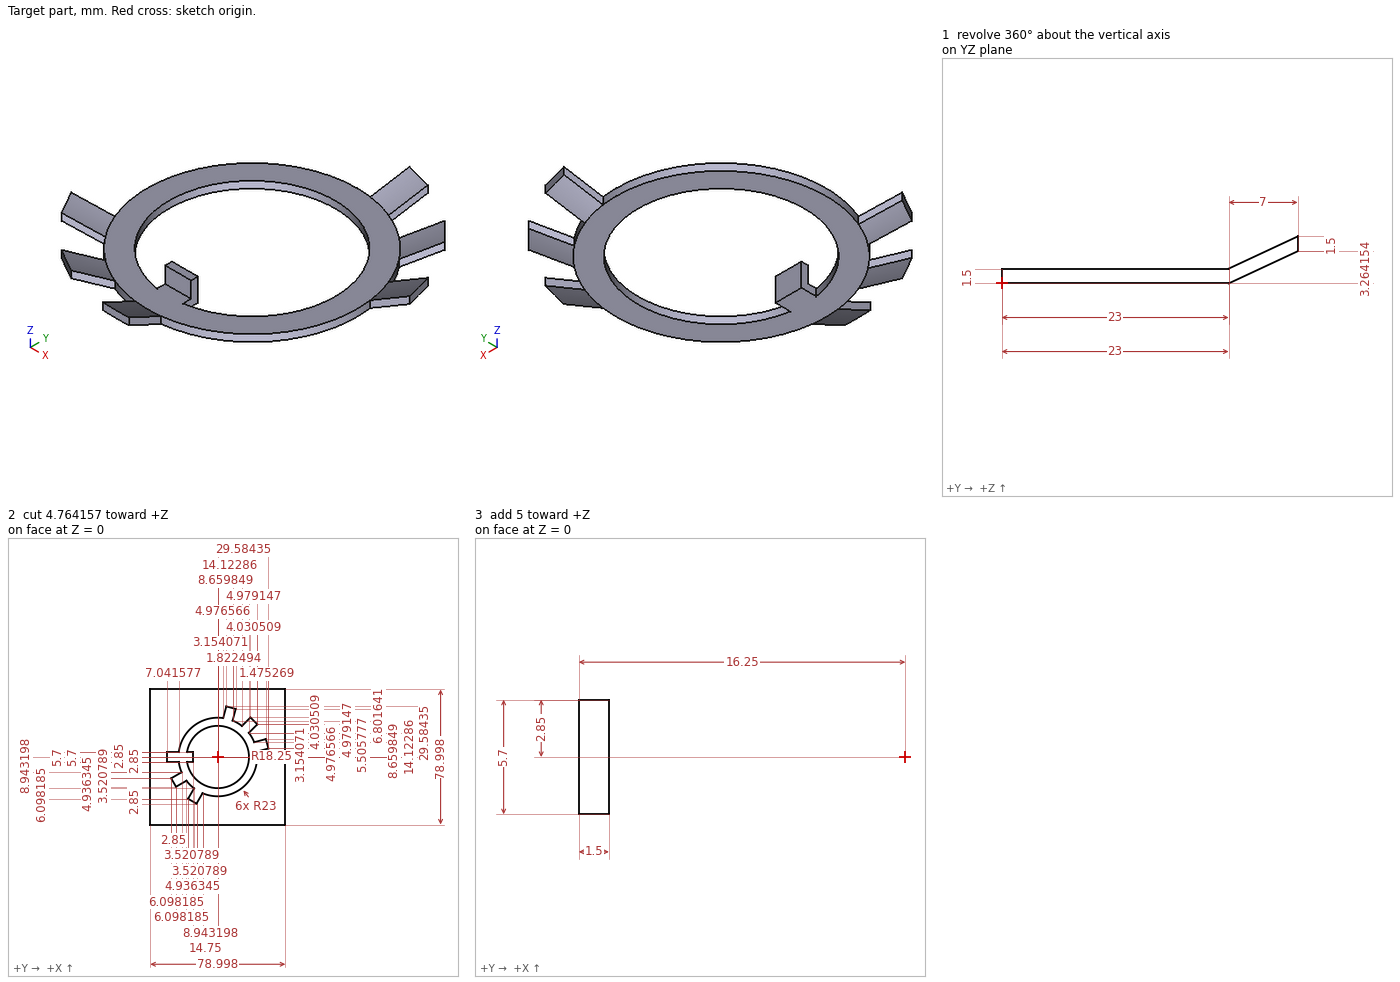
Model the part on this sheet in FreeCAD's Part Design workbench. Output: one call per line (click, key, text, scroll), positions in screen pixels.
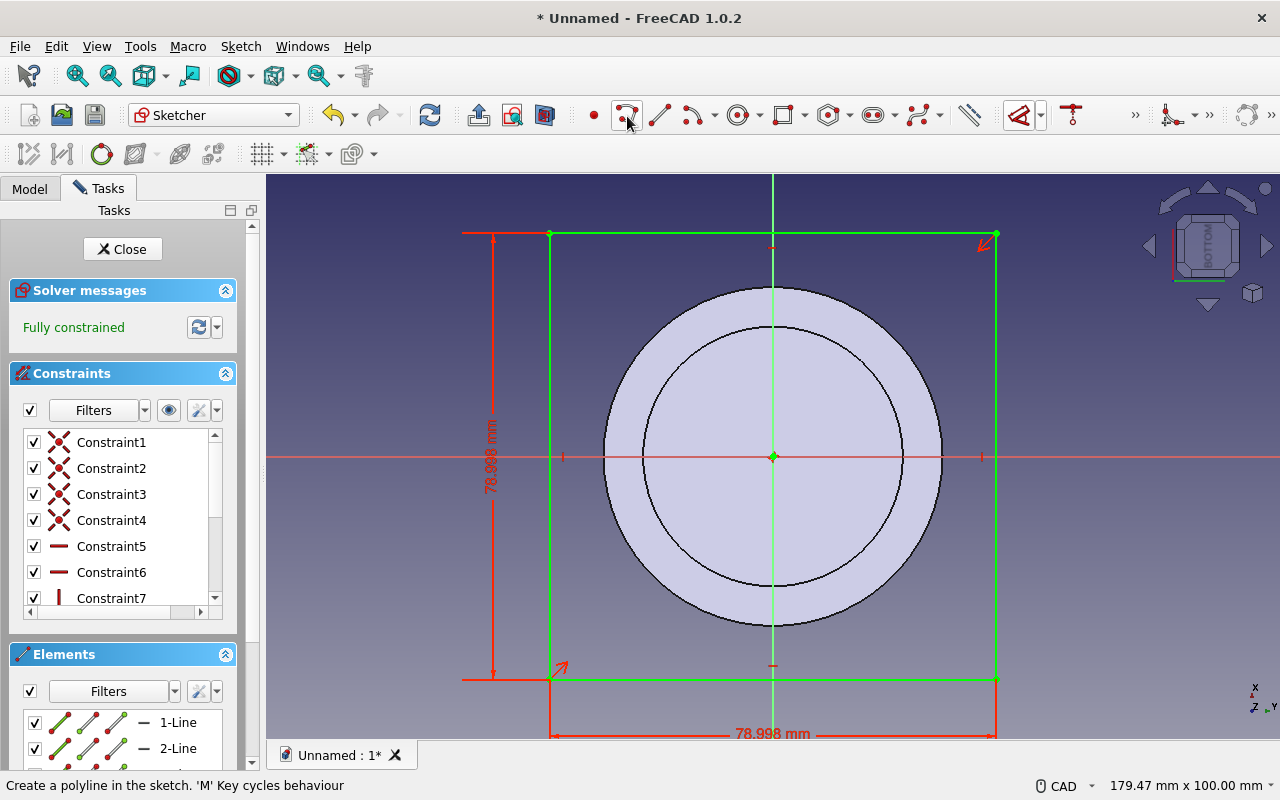
click(671, 473)
click(690, 473)
click(690, 440)
click(671, 440)
right_click(671, 440)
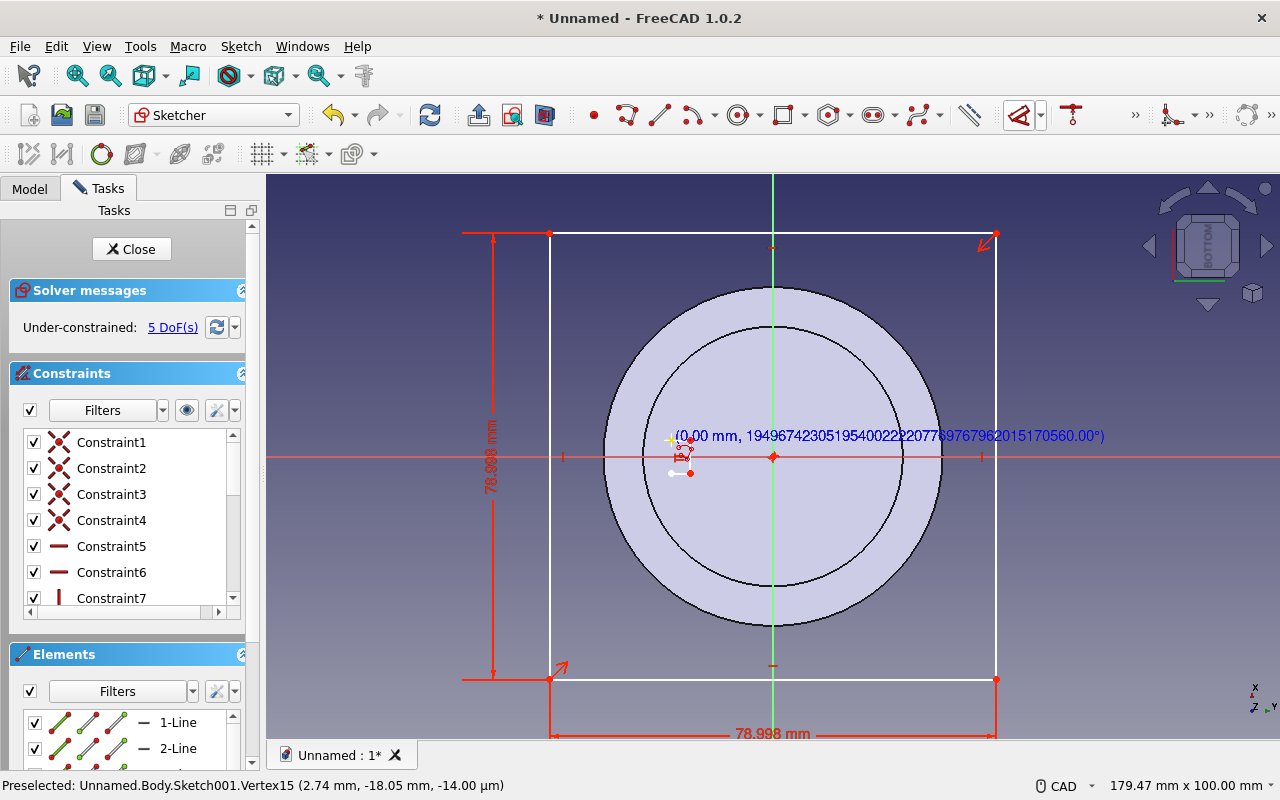
click(714, 116)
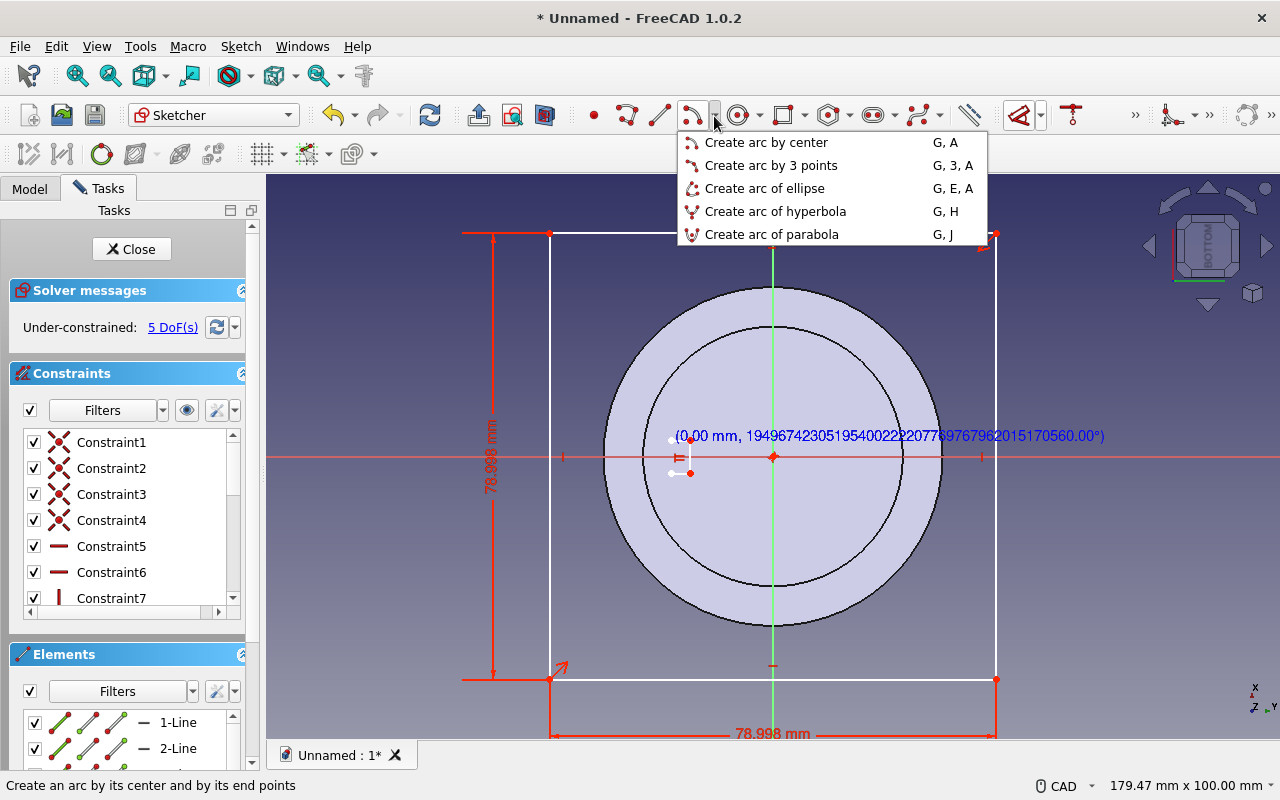
click(832, 166)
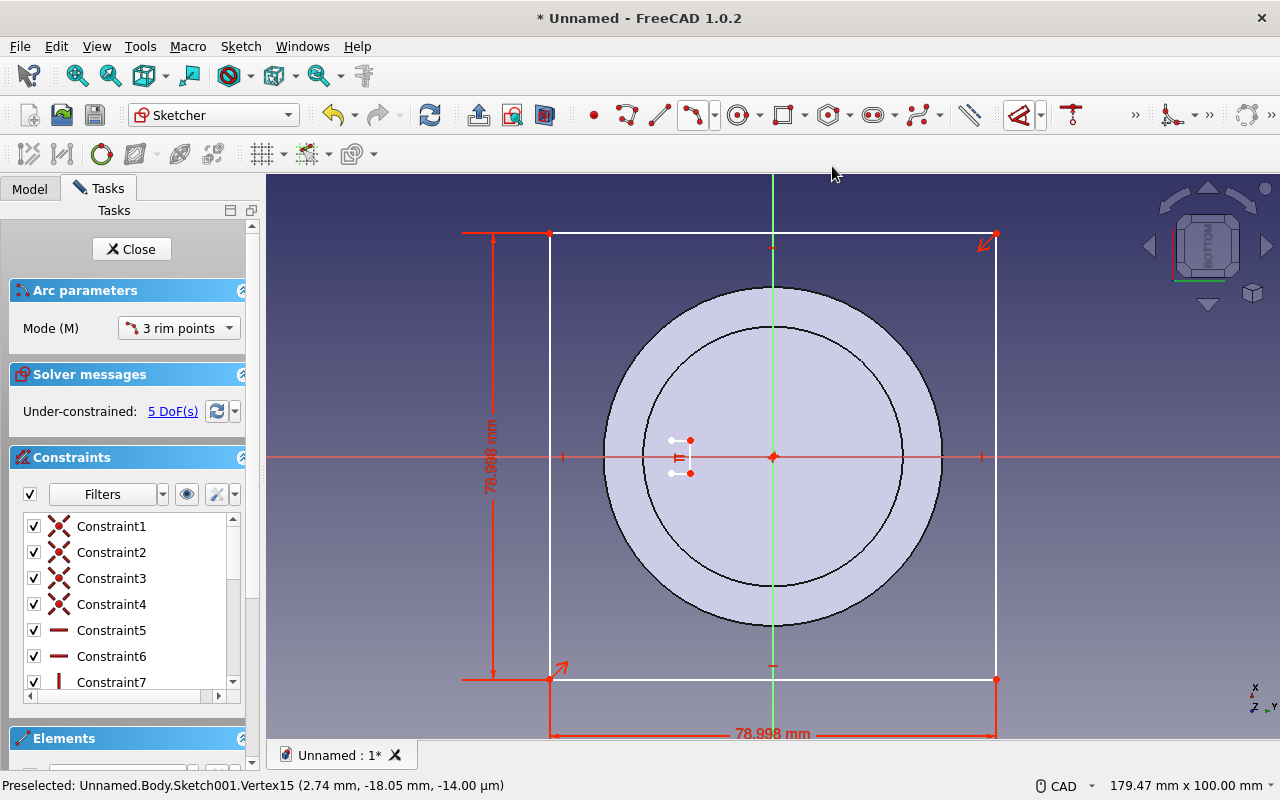
scroll(671, 440, up, 3)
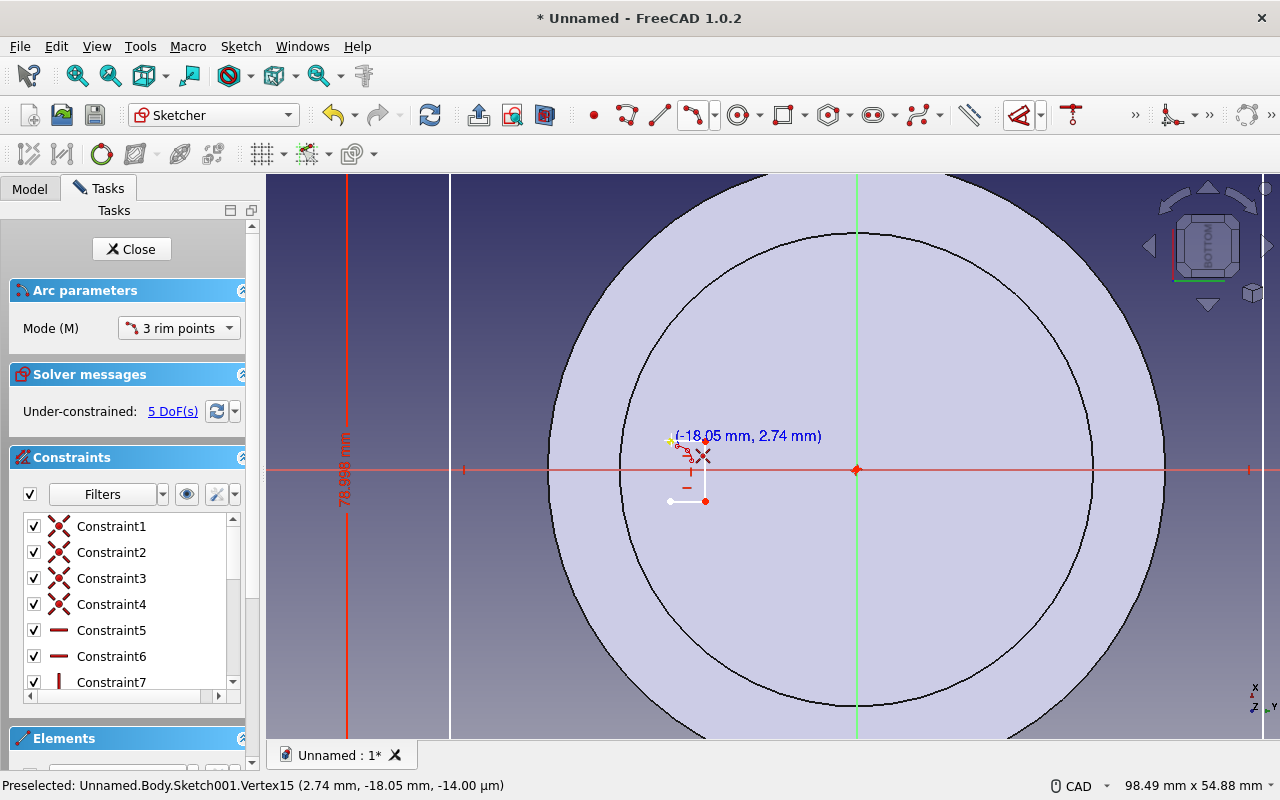
click(671, 441)
click(671, 502)
click(1012, 575)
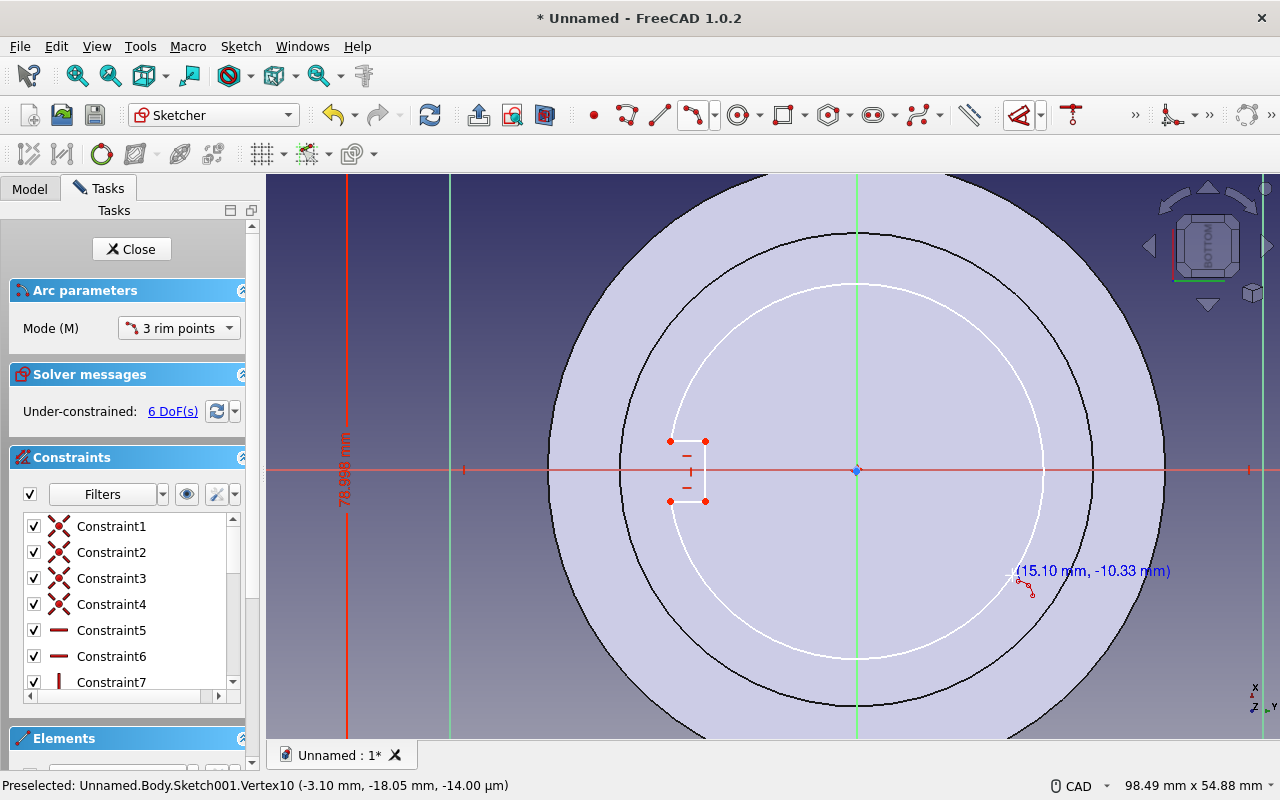
key(g)
key(m)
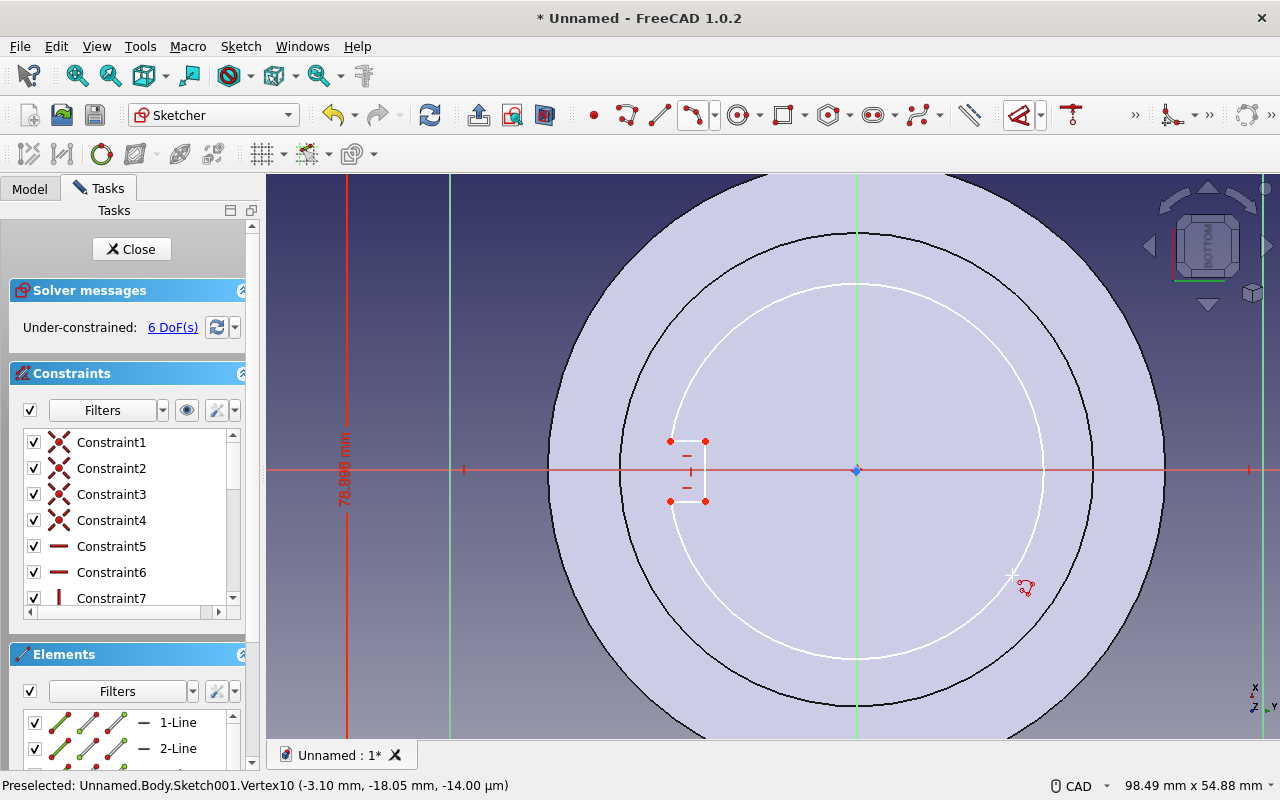
click(638, 562)
click(576, 598)
click(605, 649)
click(668, 613)
right_click(668, 613)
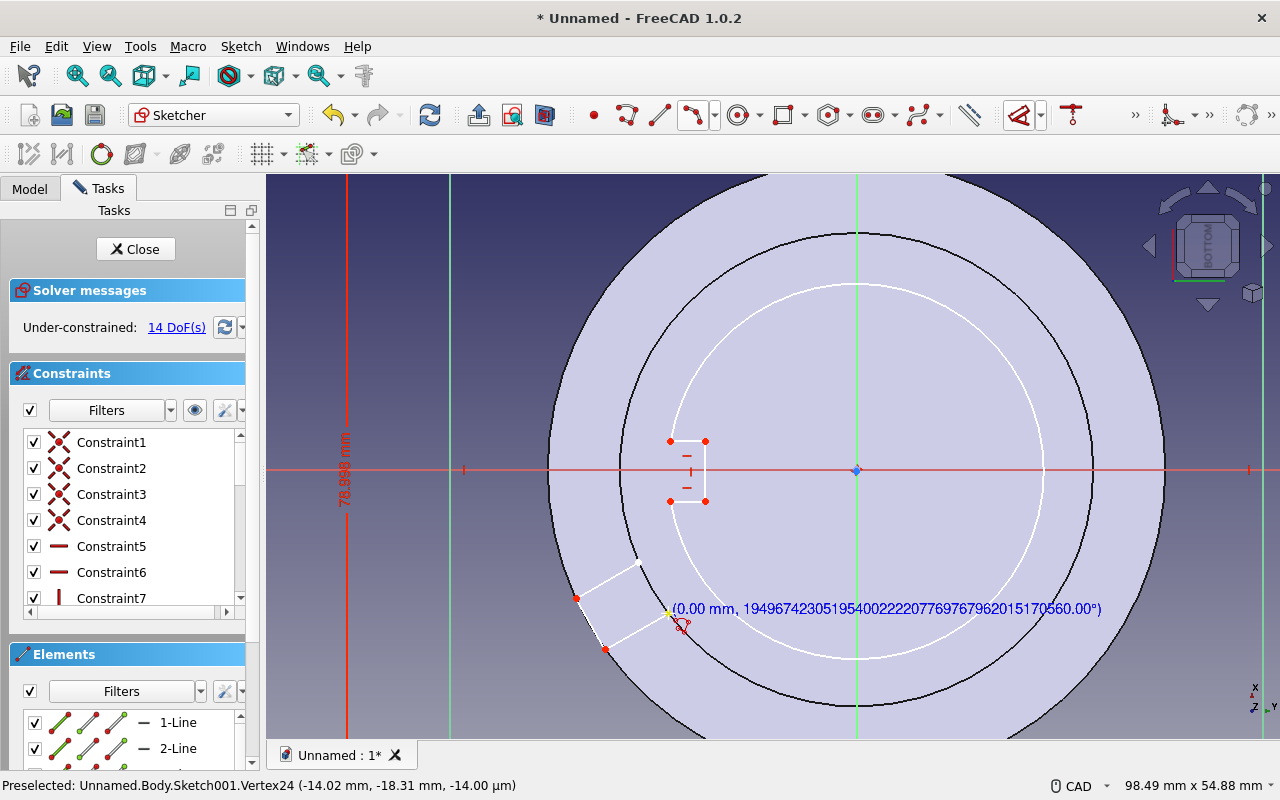
click(714, 658)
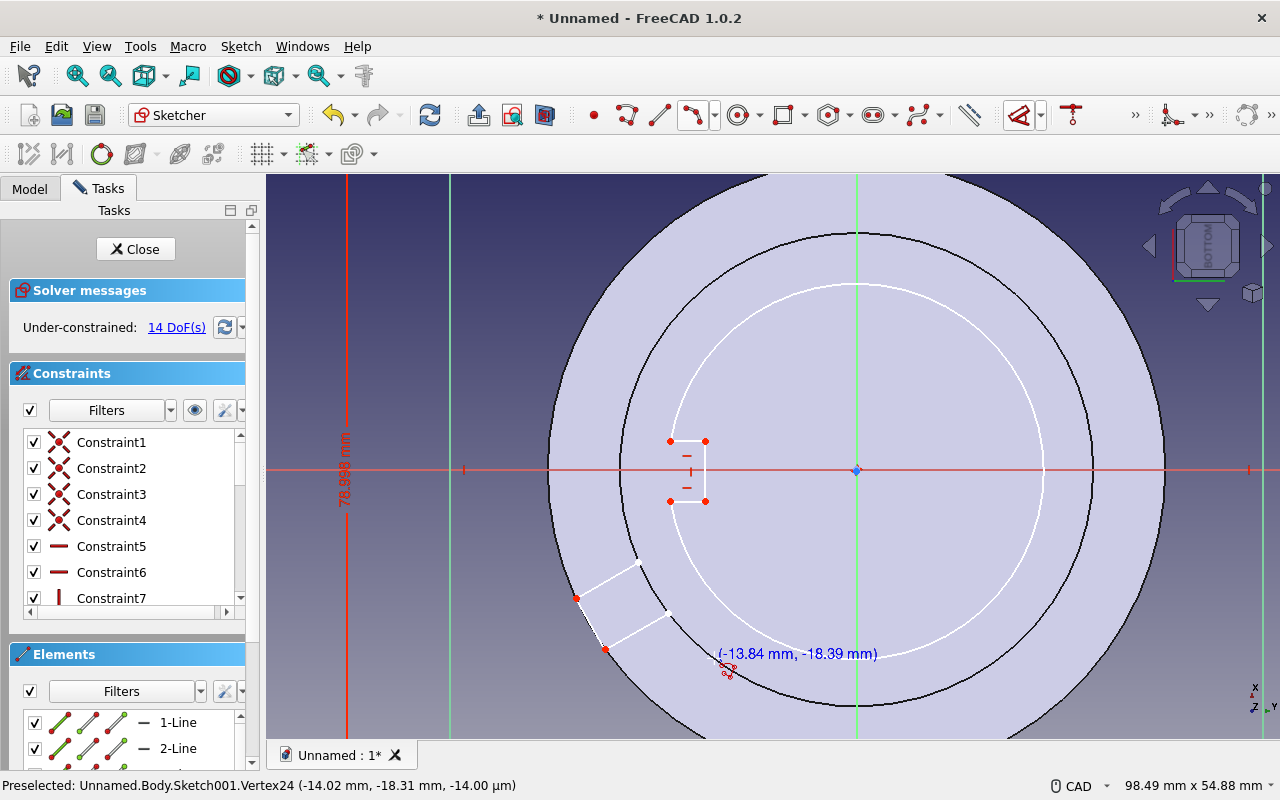
scroll(580, 446, down, 4)